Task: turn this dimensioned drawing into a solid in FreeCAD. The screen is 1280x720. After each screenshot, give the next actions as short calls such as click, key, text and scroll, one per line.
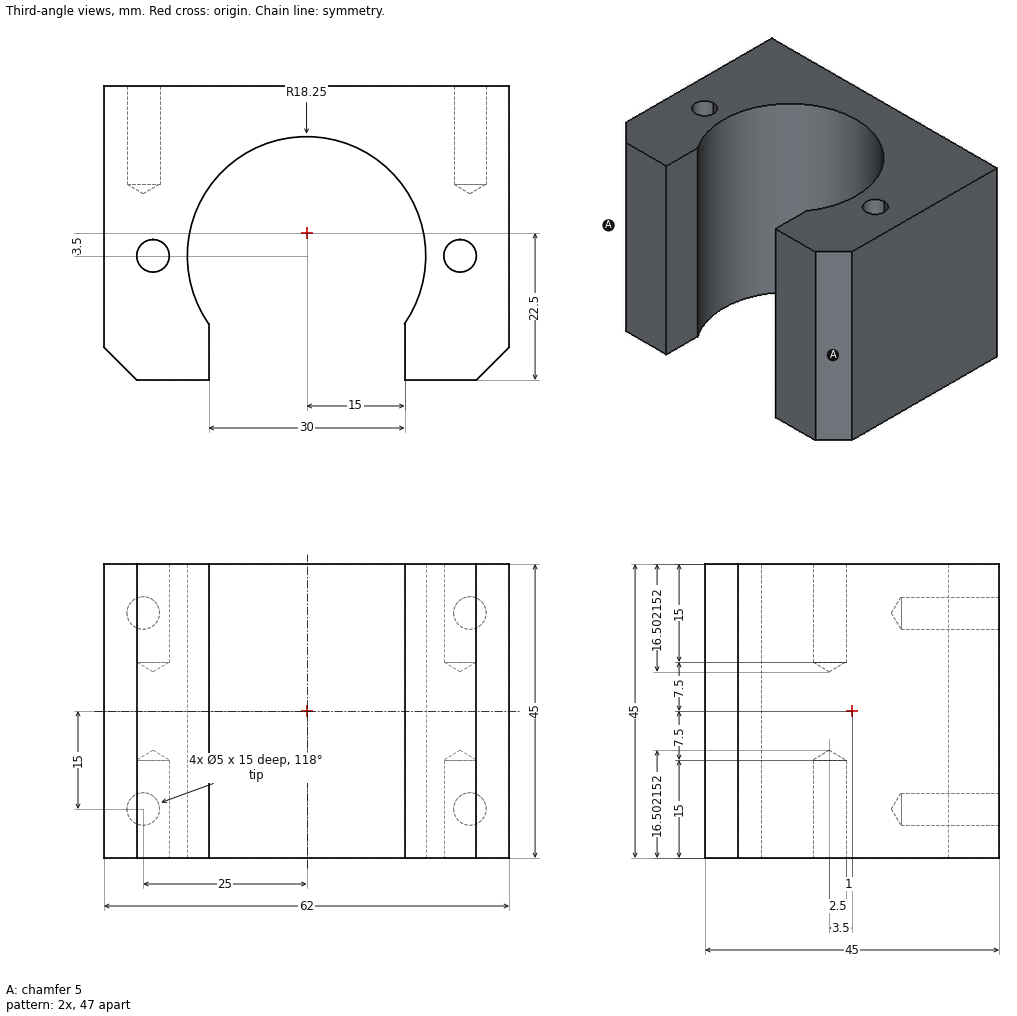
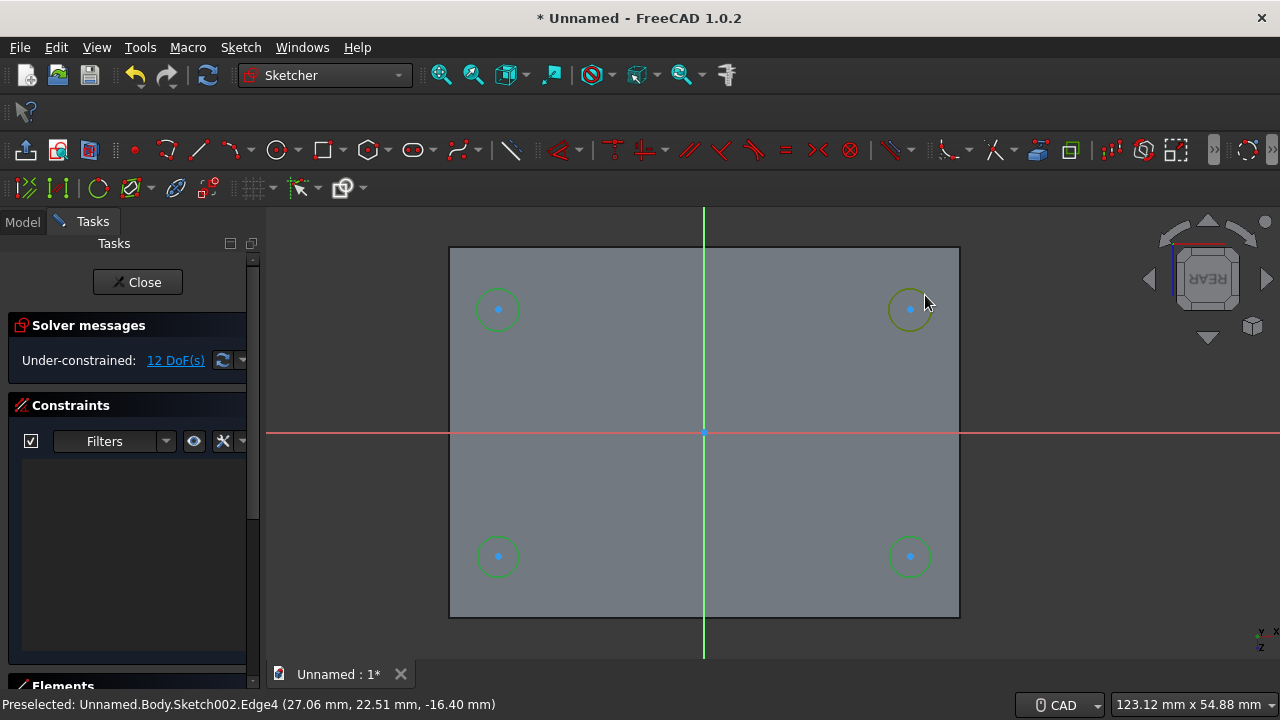
click(786, 150)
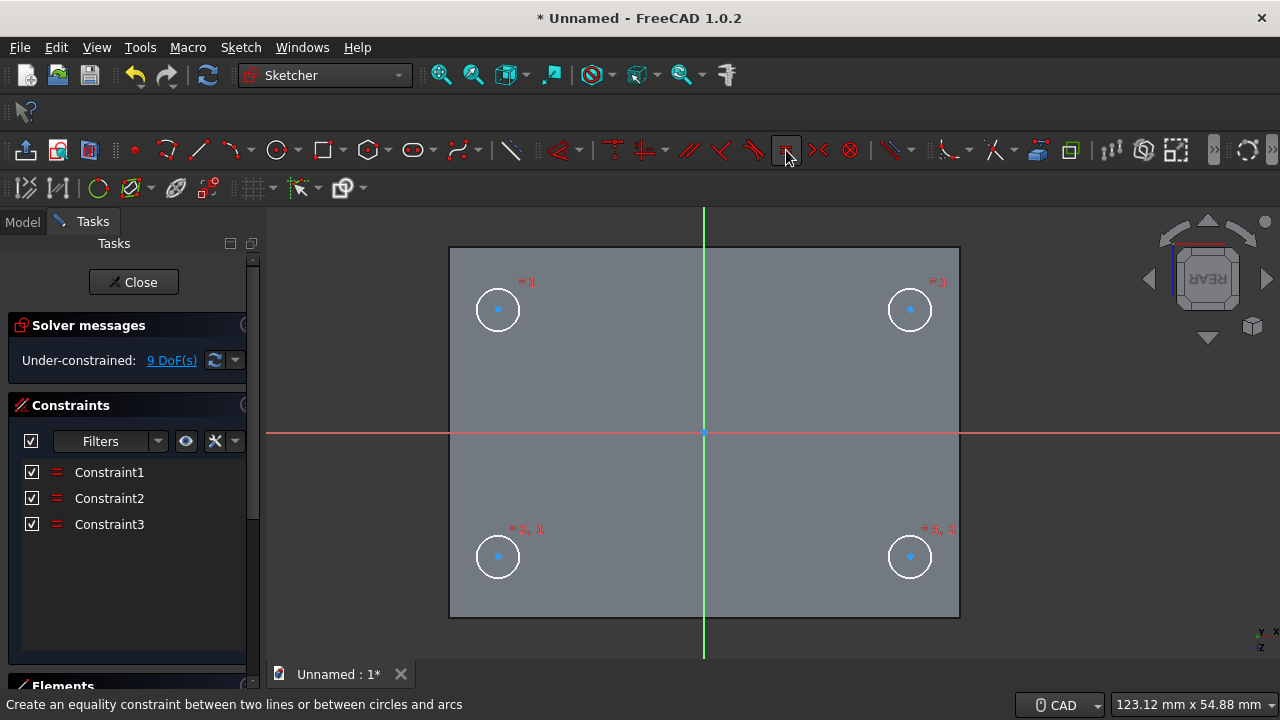
click(498, 310)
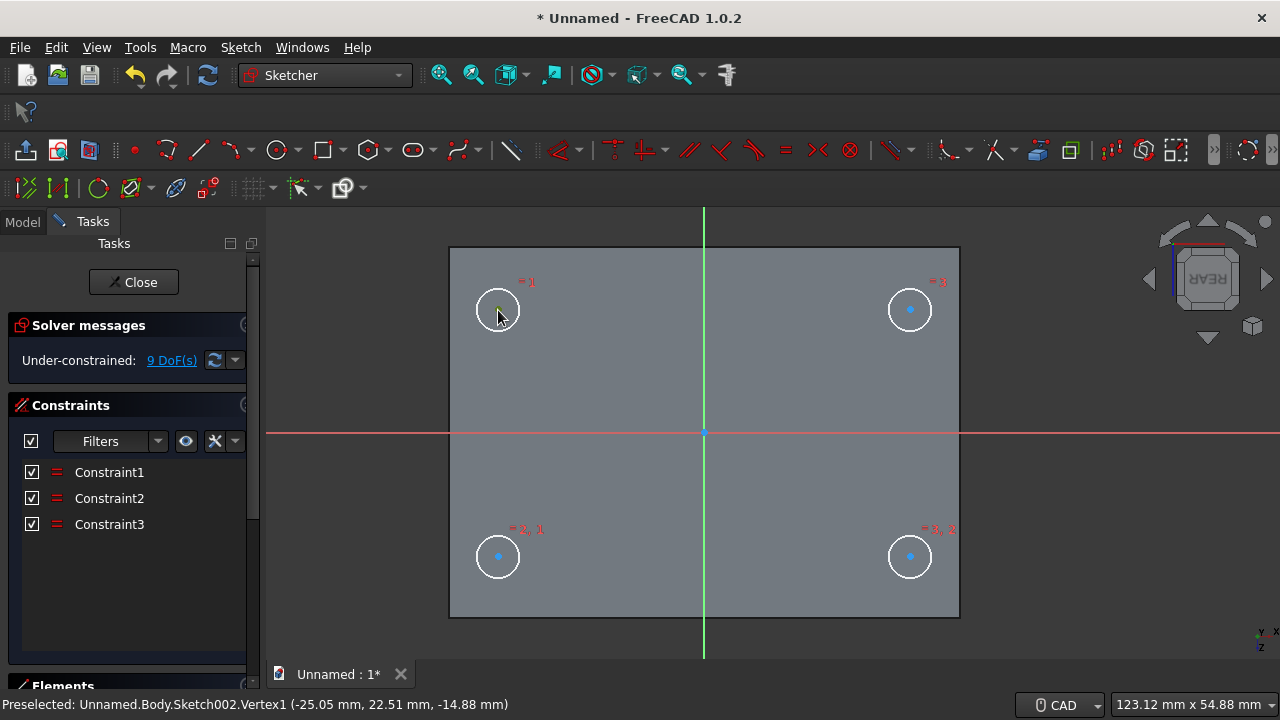
click(498, 557)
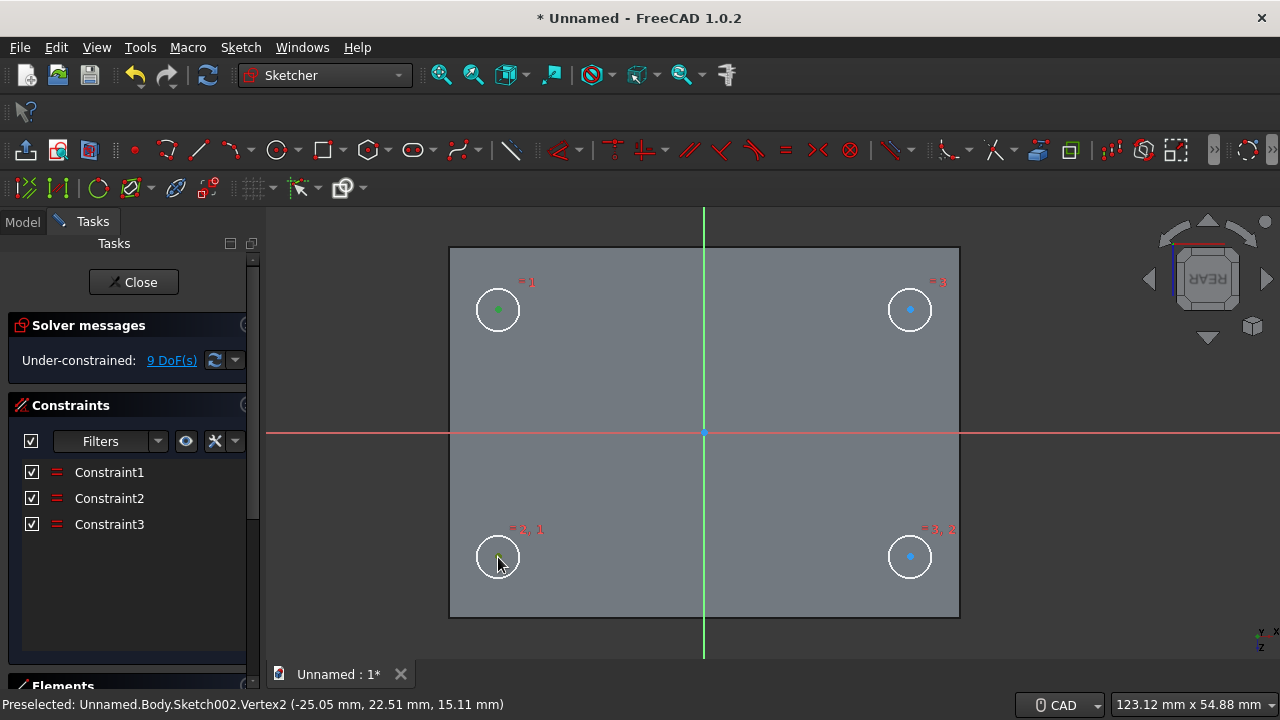
click(353, 433)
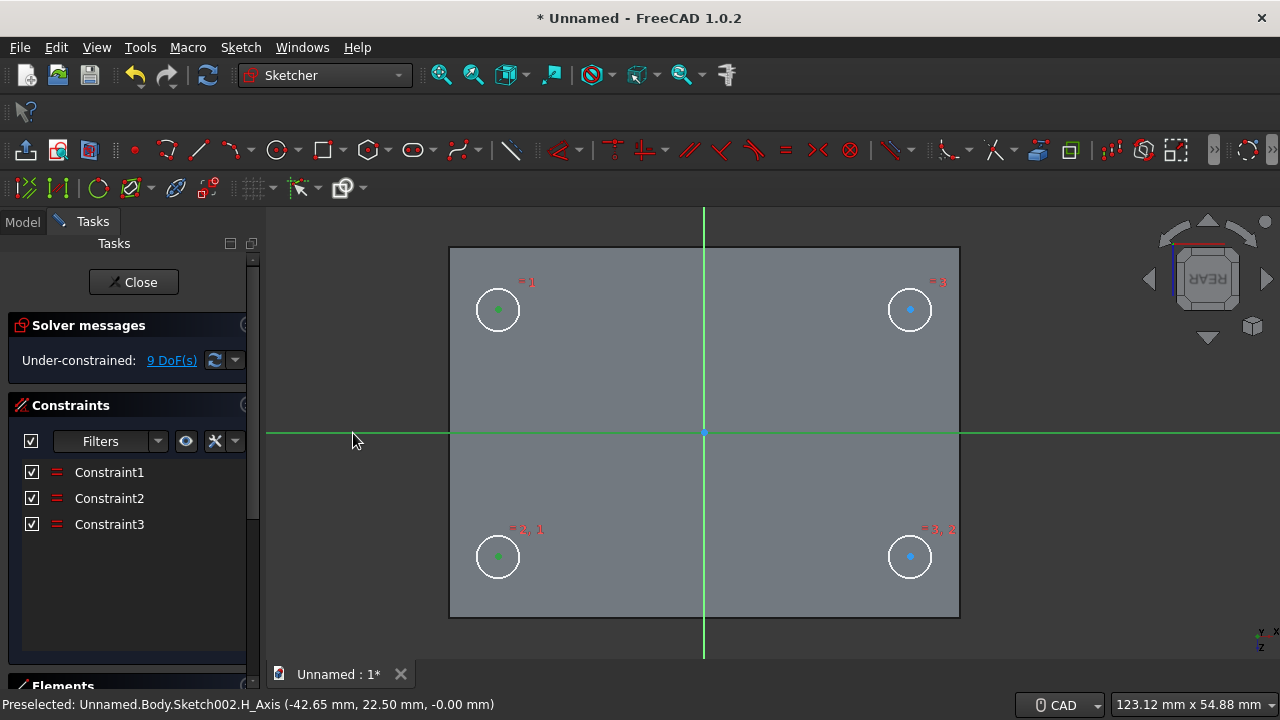
click(818, 150)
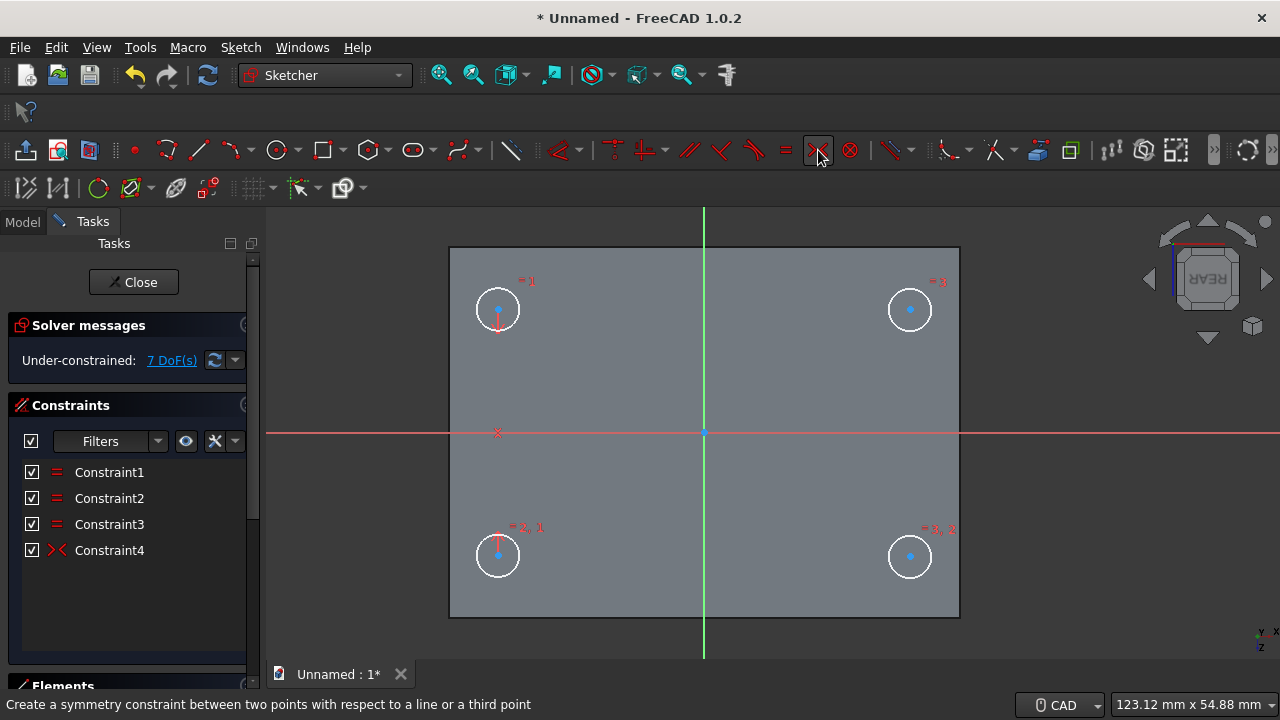
click(498, 556)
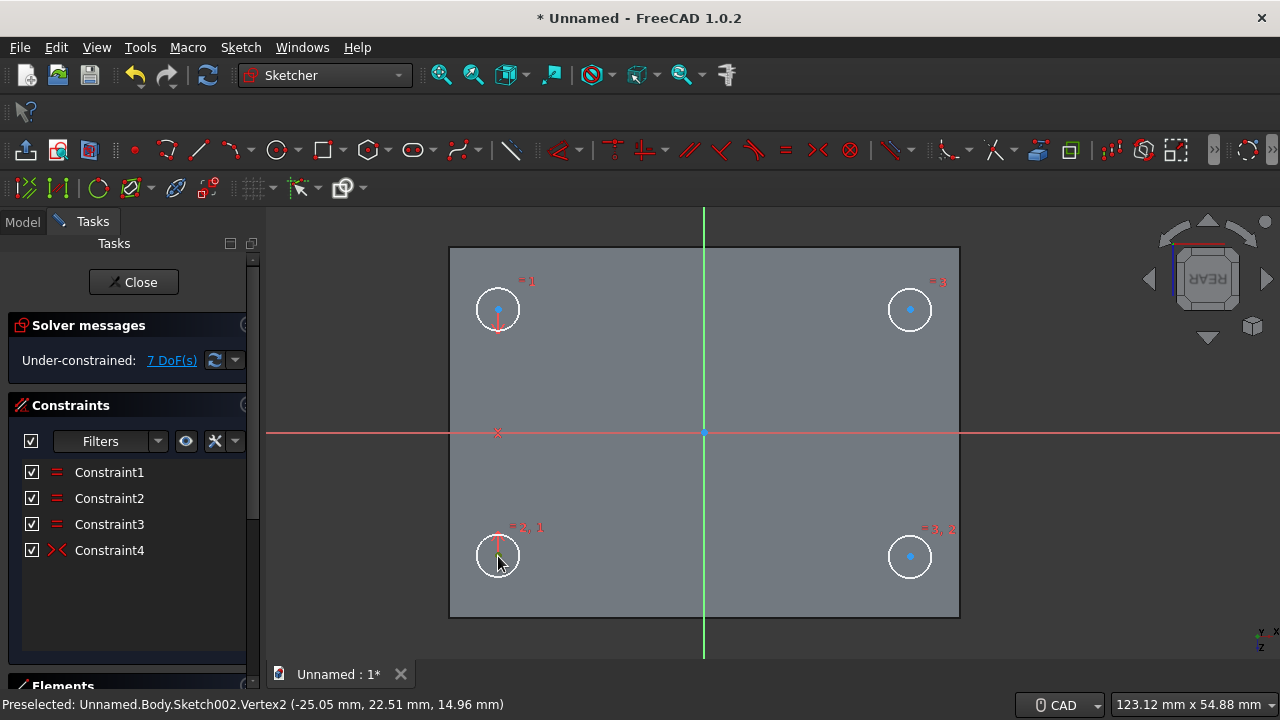
click(910, 557)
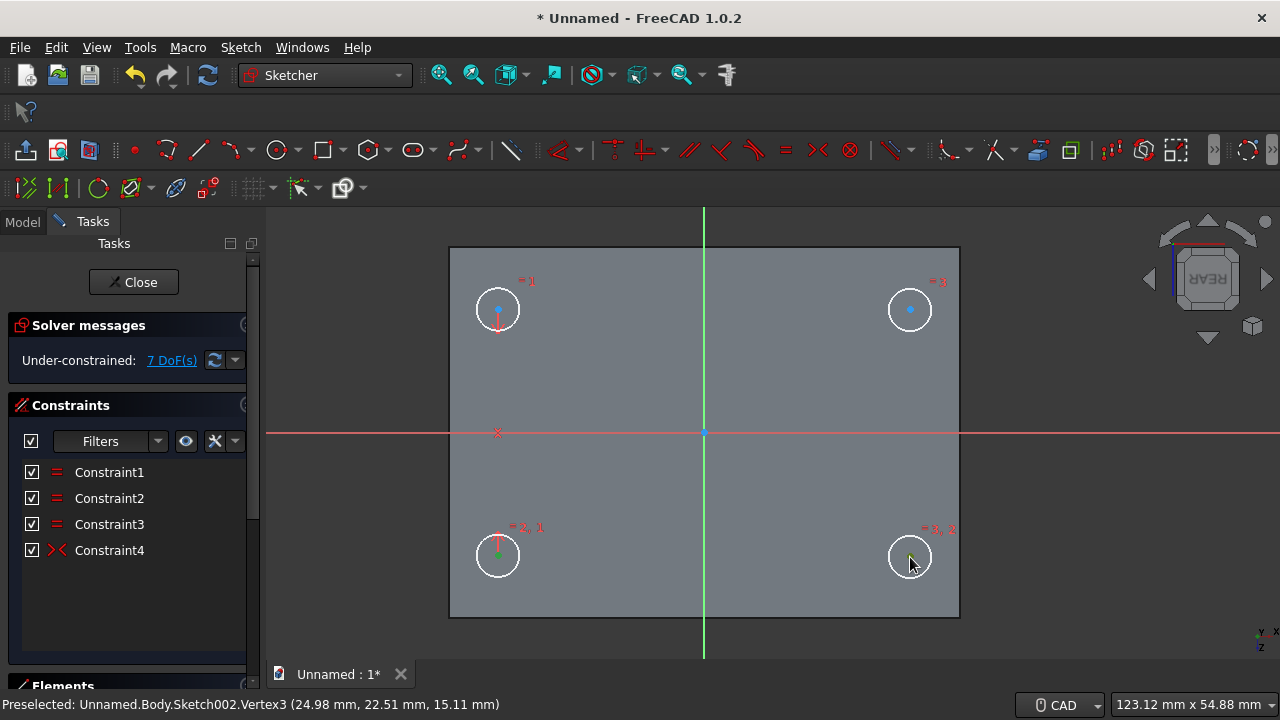
click(704, 603)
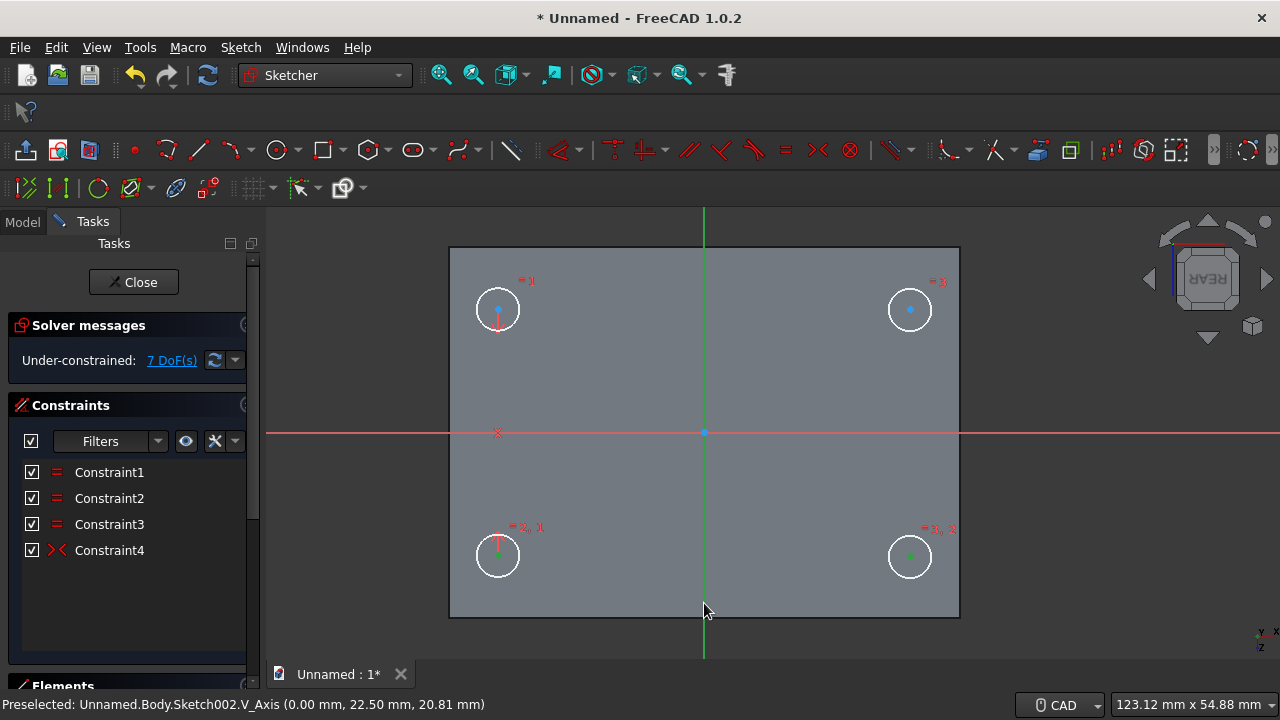
click(818, 150)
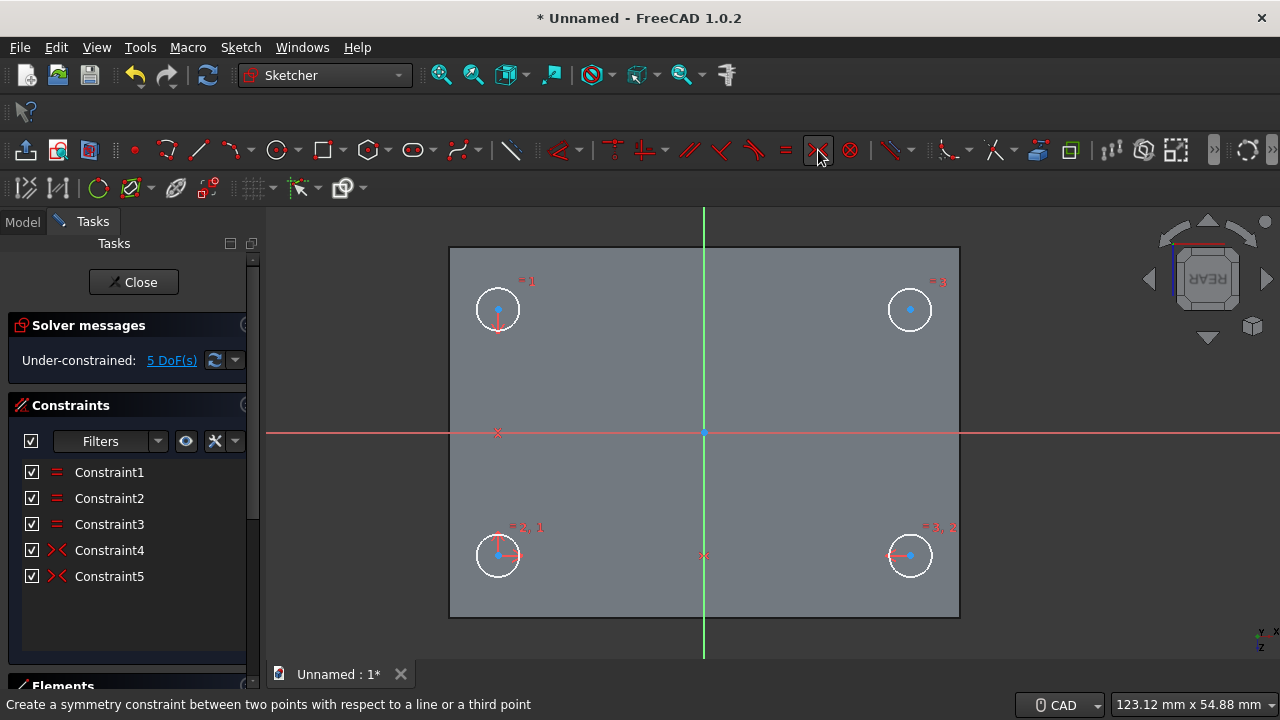
click(498, 309)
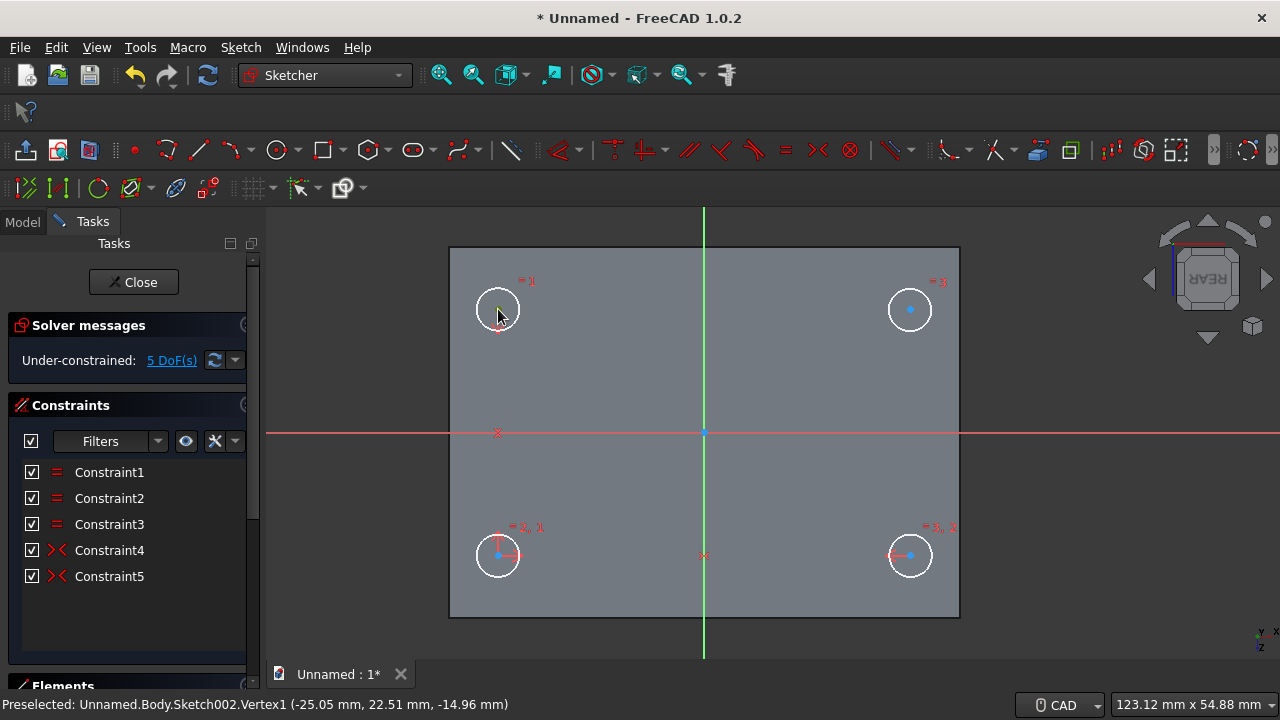
click(910, 310)